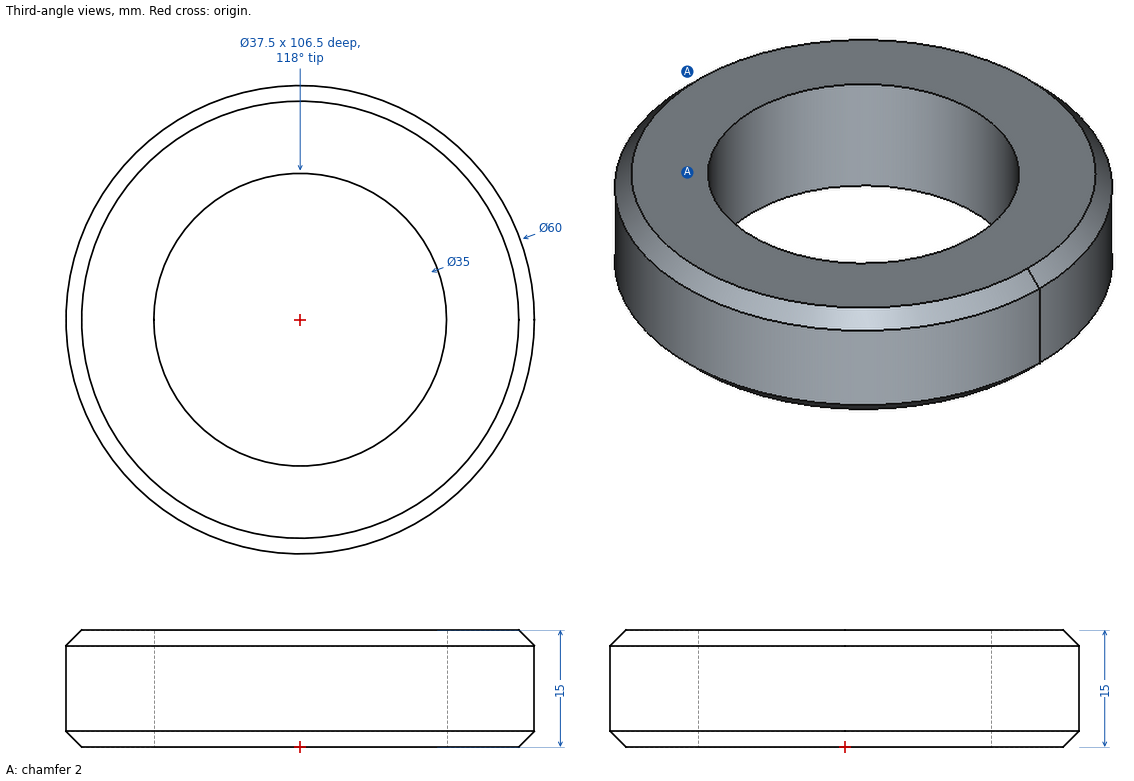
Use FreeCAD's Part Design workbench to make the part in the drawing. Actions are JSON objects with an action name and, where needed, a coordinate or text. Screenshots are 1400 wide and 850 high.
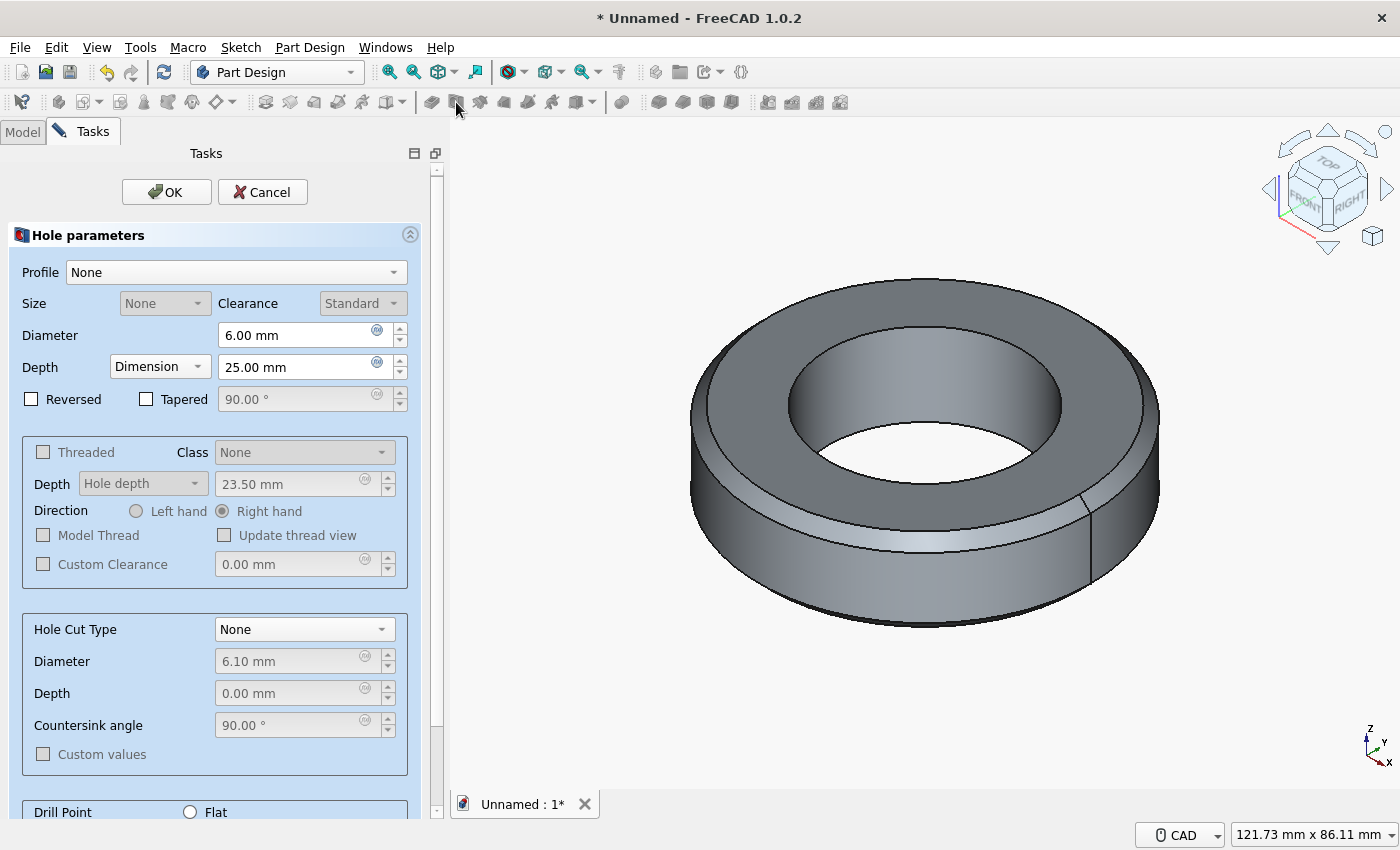
{"action": "triple_click", "coordinate": [305, 335]}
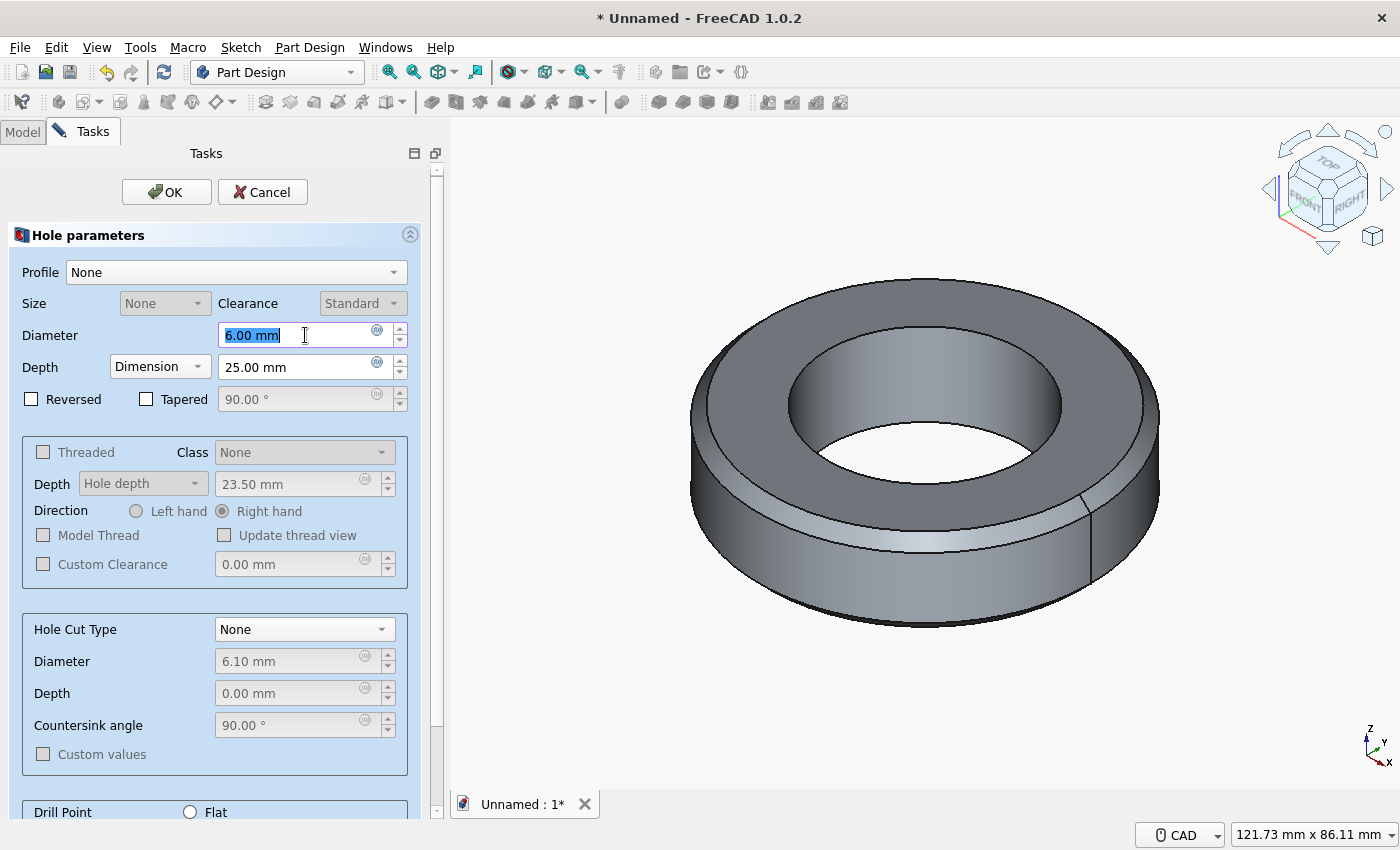
{"action": "type", "text": "37.5"}
{"action": "key", "text": "Tab"}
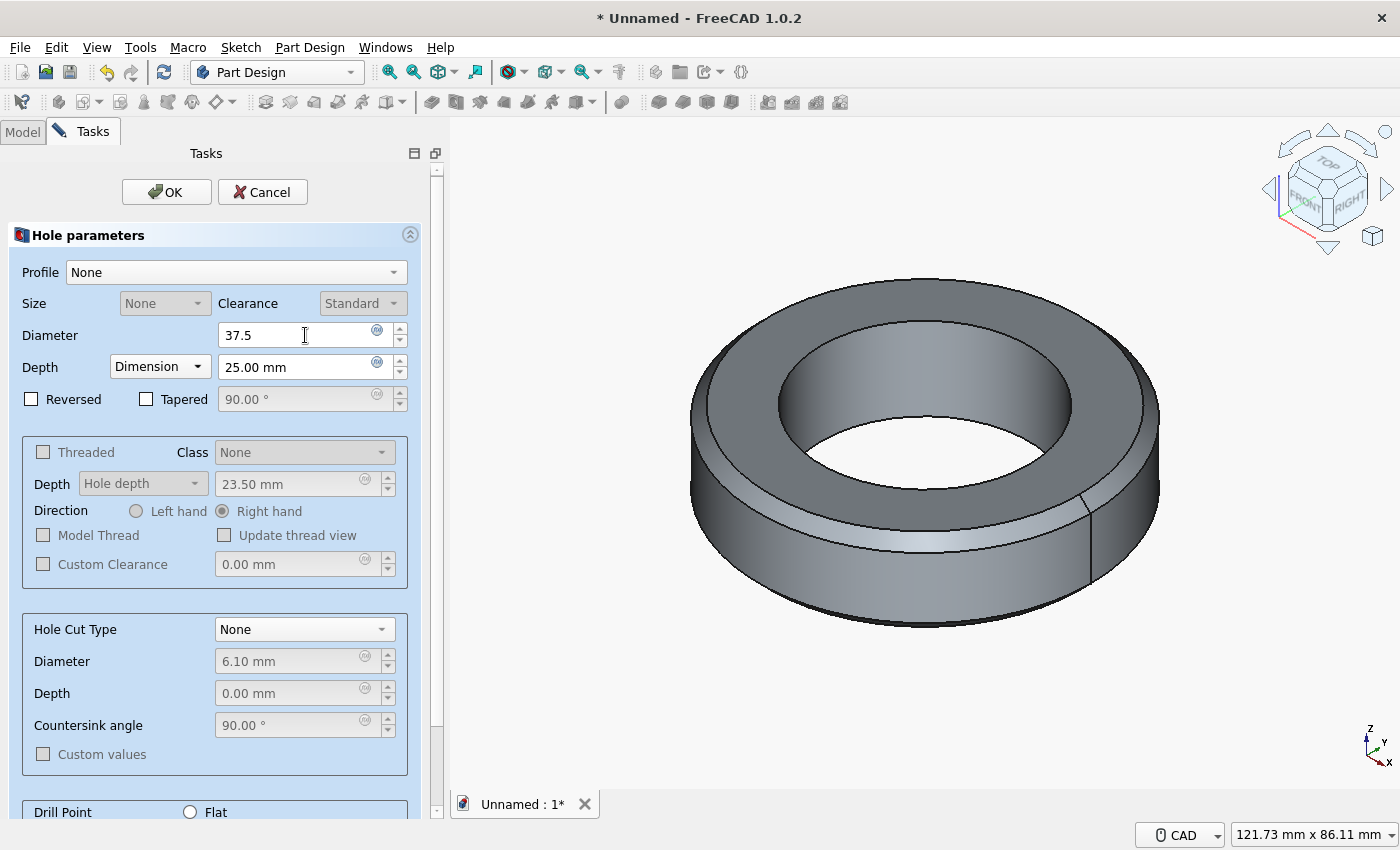
{"action": "triple_click", "coordinate": [305, 367]}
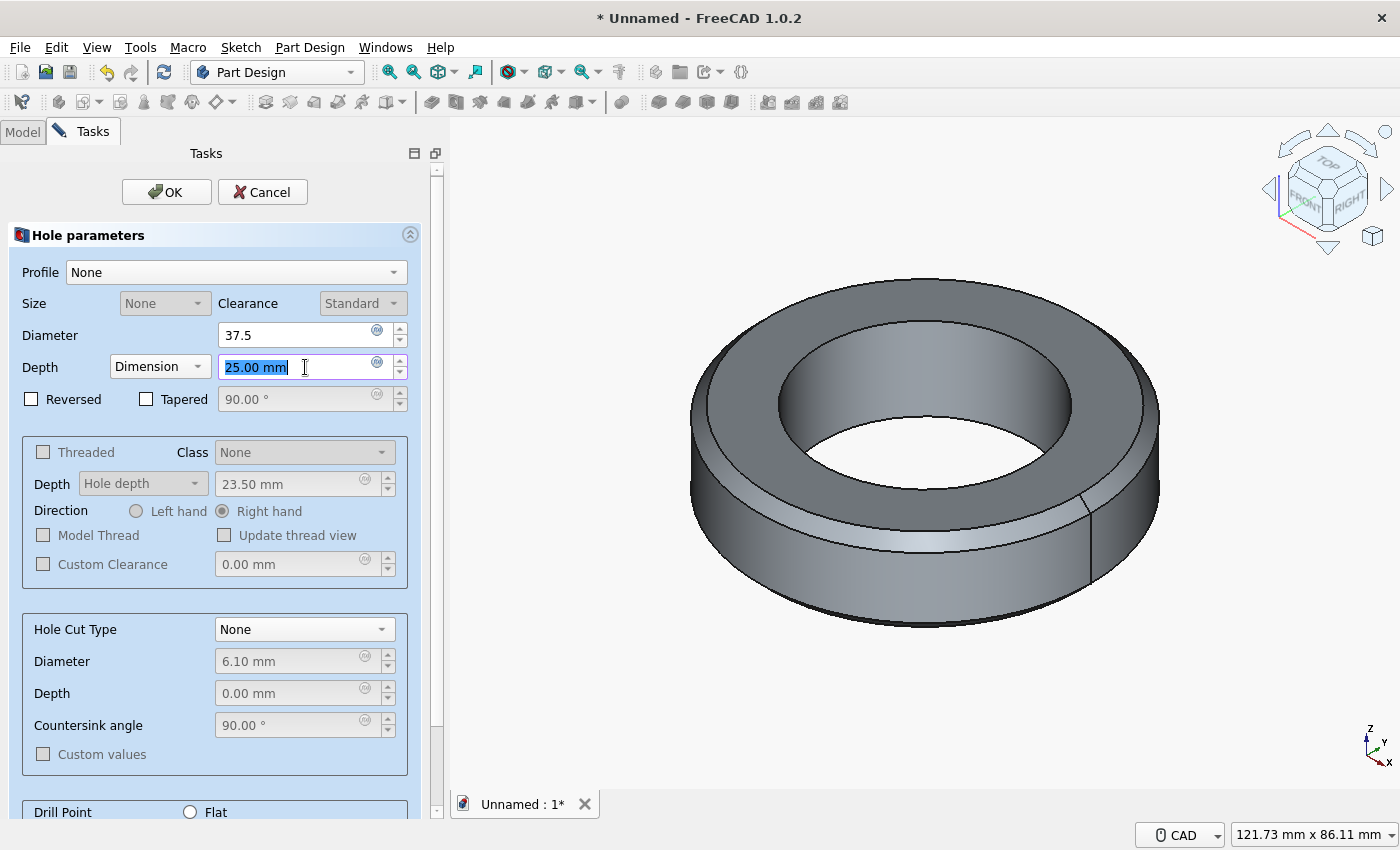
{"action": "type", "text": "106.5"}
{"action": "key", "text": "Tab"}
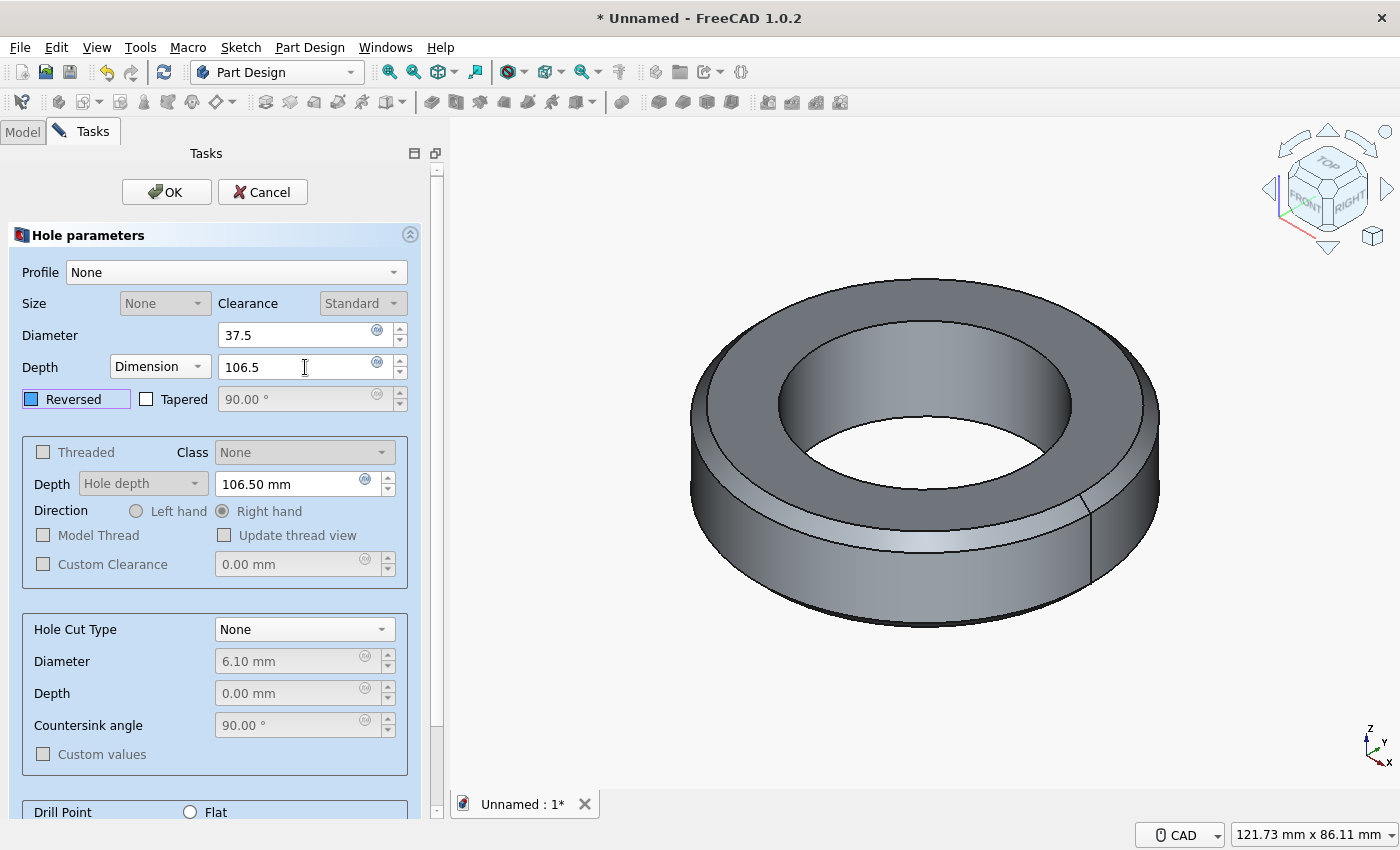
{"action": "left_click", "coordinate": [167, 192]}